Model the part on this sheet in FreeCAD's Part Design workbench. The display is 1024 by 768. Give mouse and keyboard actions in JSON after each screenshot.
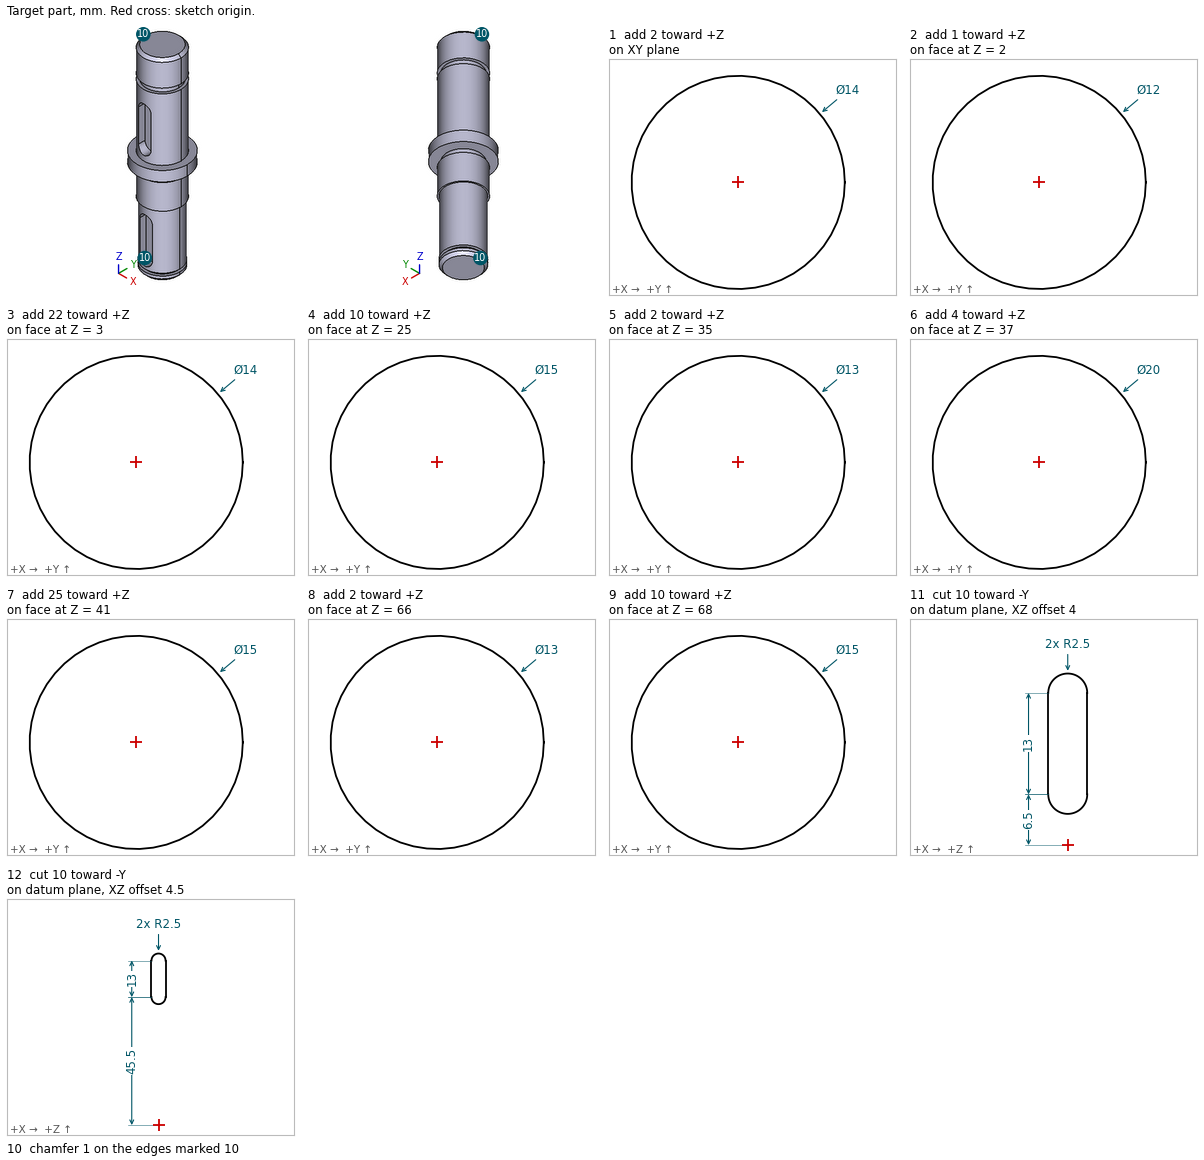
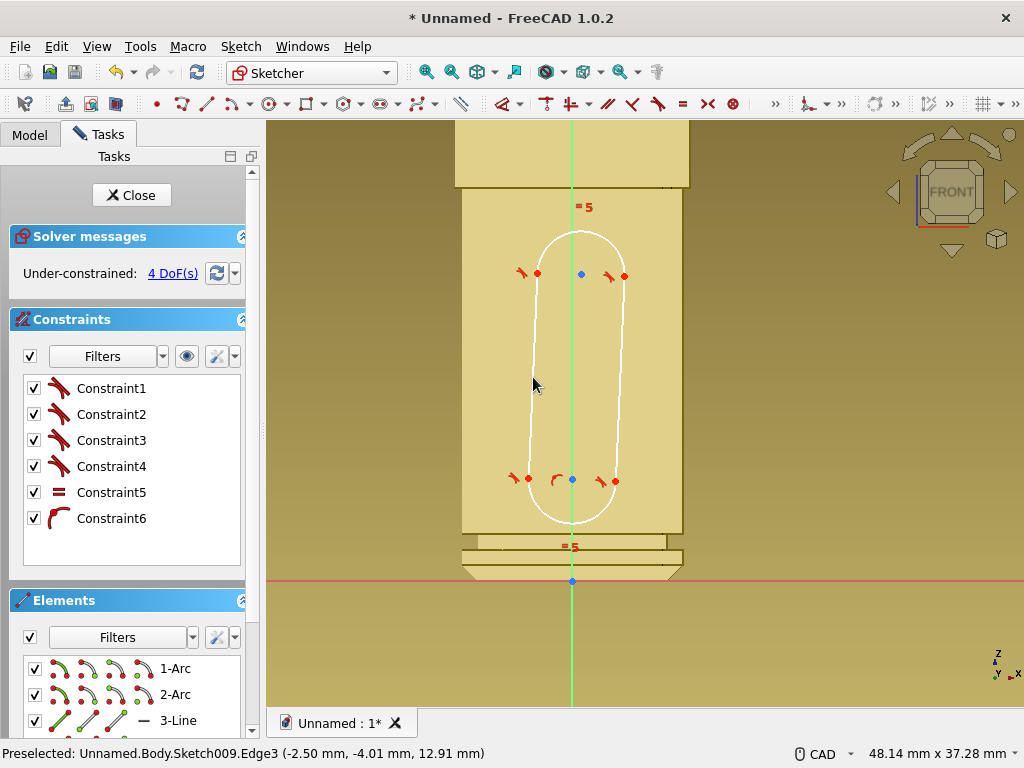
{"action": "left_click", "coordinate": [531, 417]}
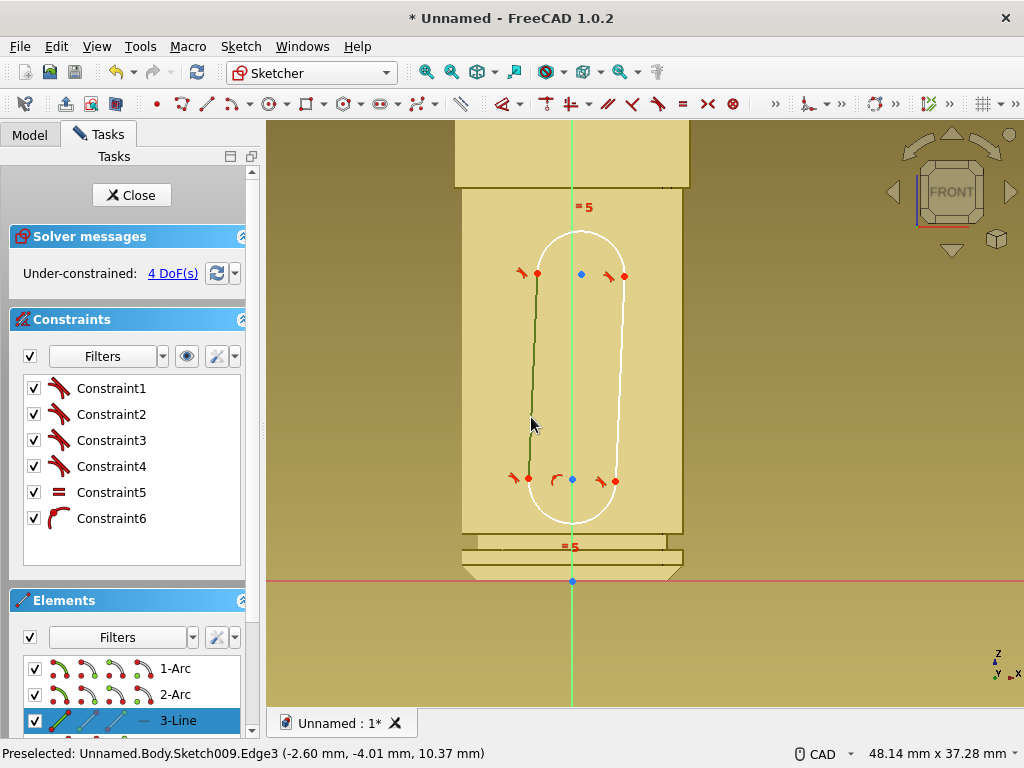
{"action": "left_click", "coordinate": [588, 104]}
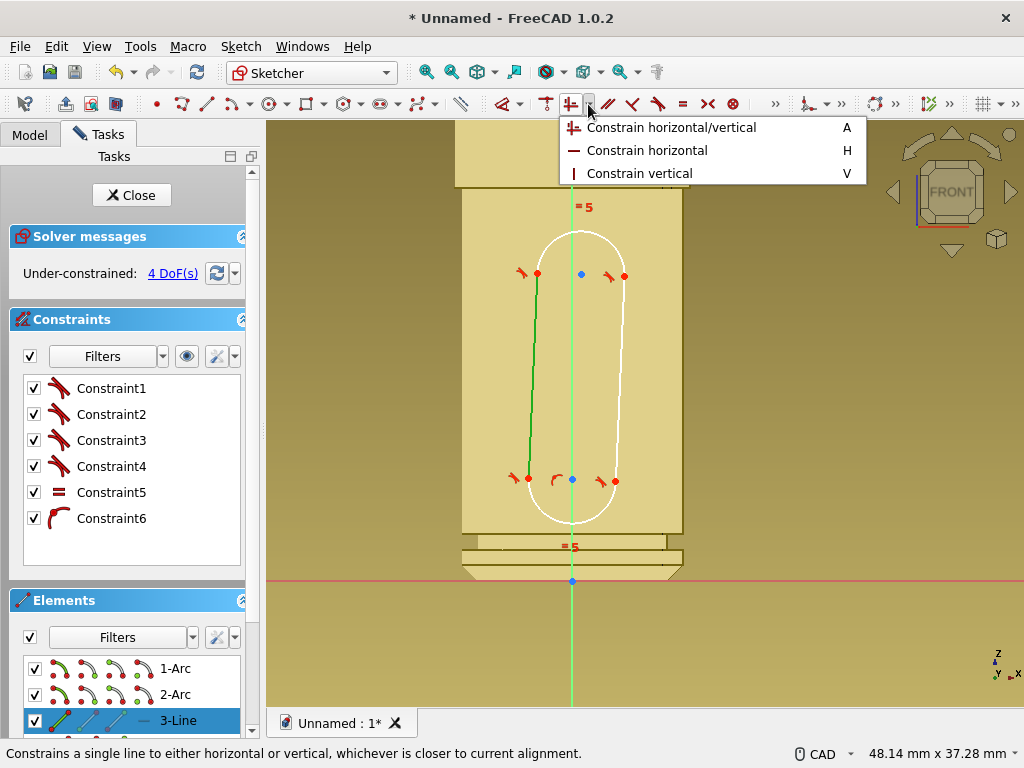
{"action": "left_click", "coordinate": [713, 174]}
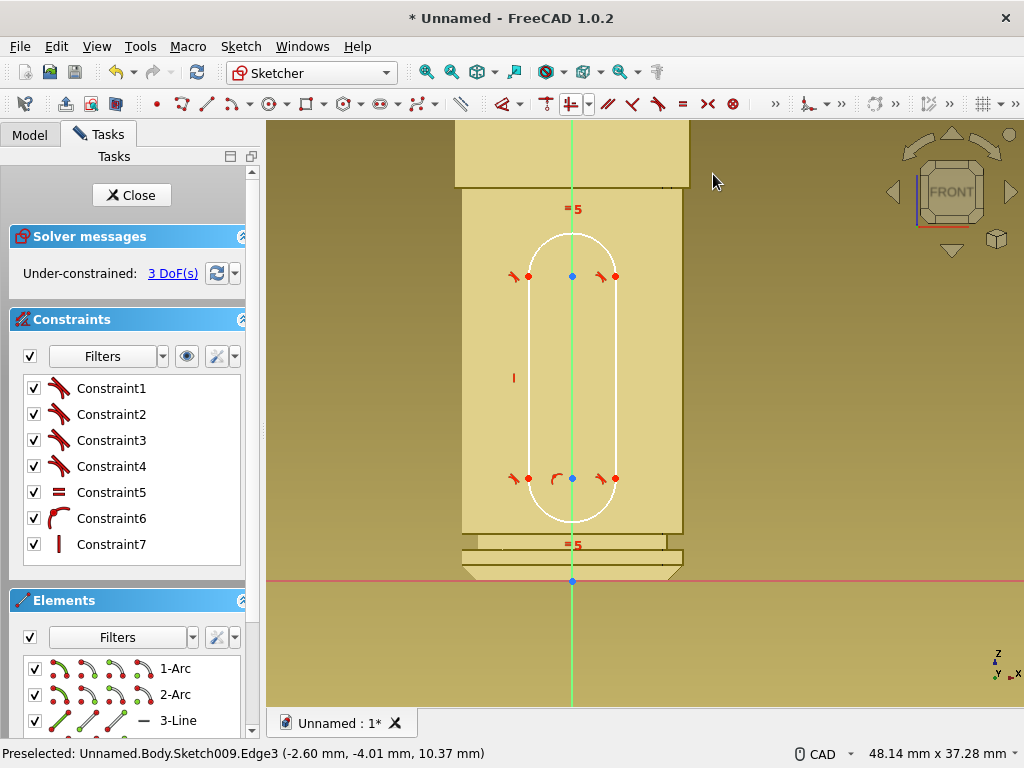
{"action": "left_click", "coordinate": [502, 104]}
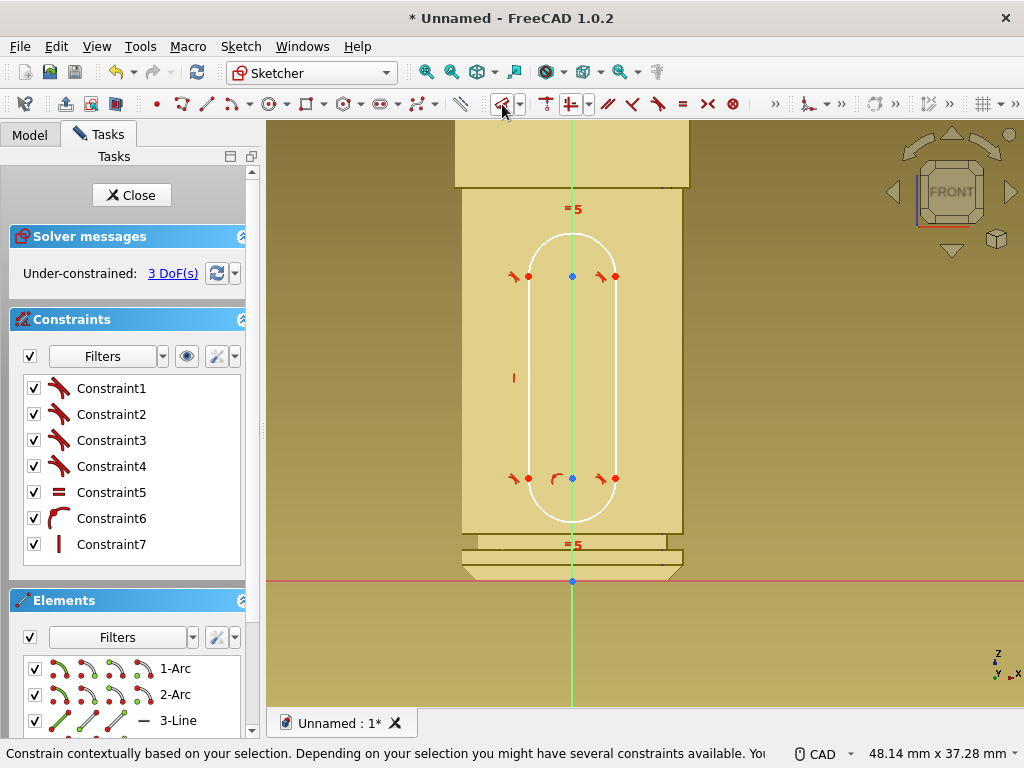
{"action": "left_click", "coordinate": [547, 514]}
{"action": "left_click", "coordinate": [528, 540]}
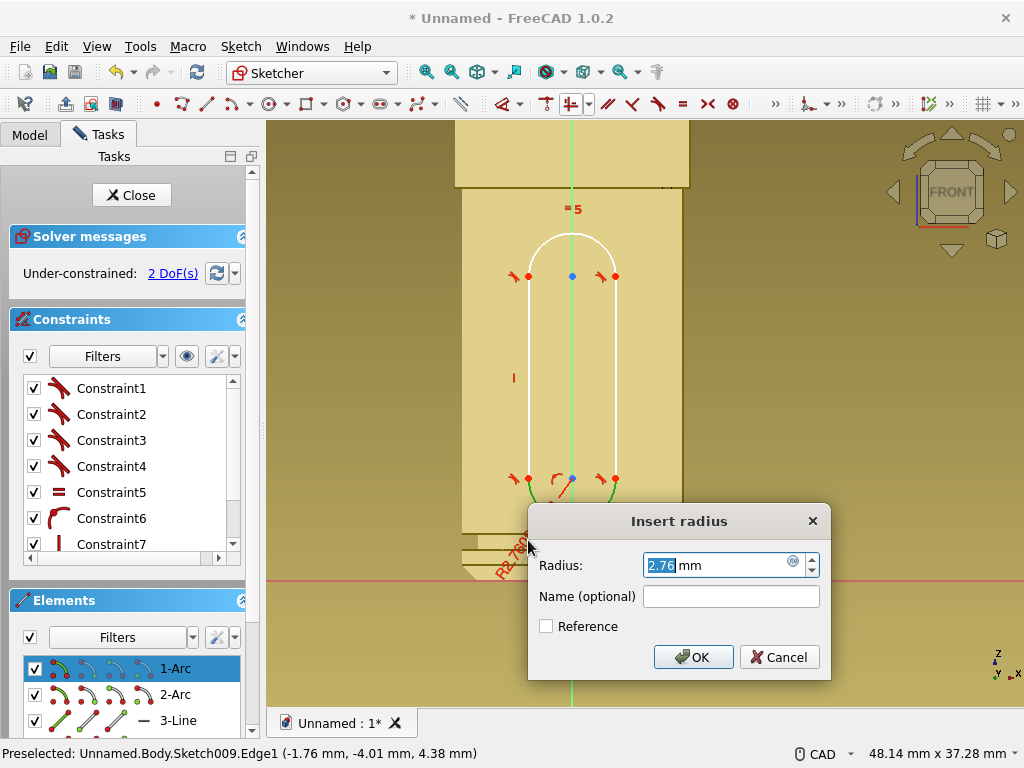
{"action": "type", "text": "2.5"}
{"action": "key", "text": "Return"}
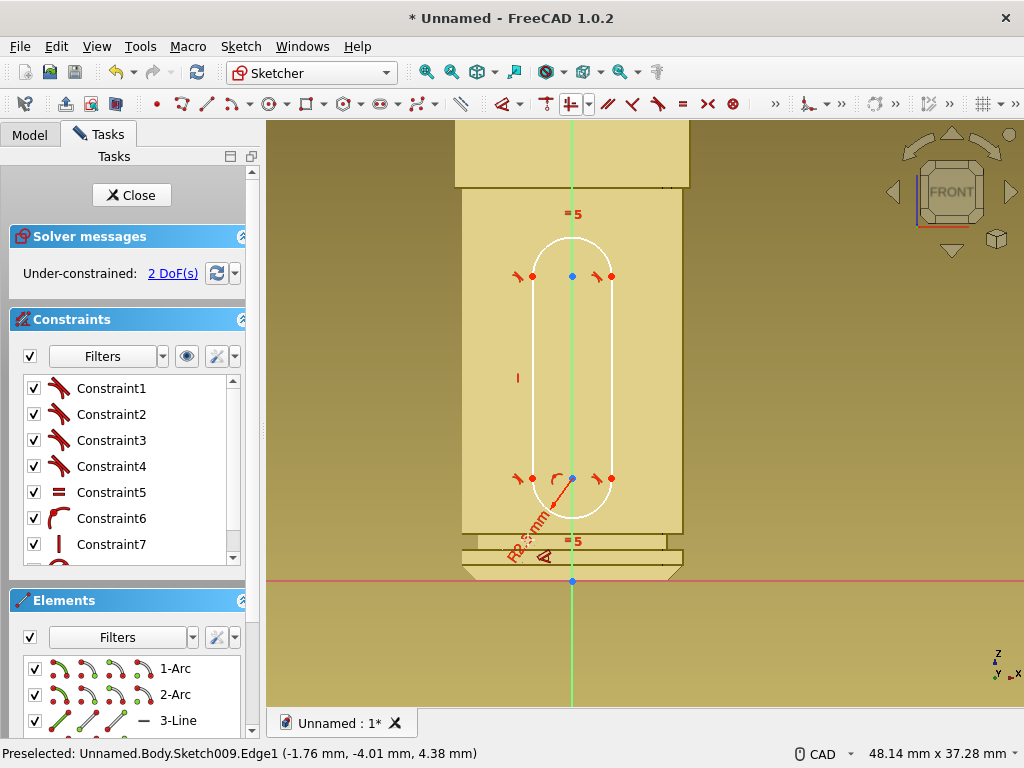
{"action": "left_click", "coordinate": [533, 418]}
{"action": "left_click", "coordinate": [499, 378]}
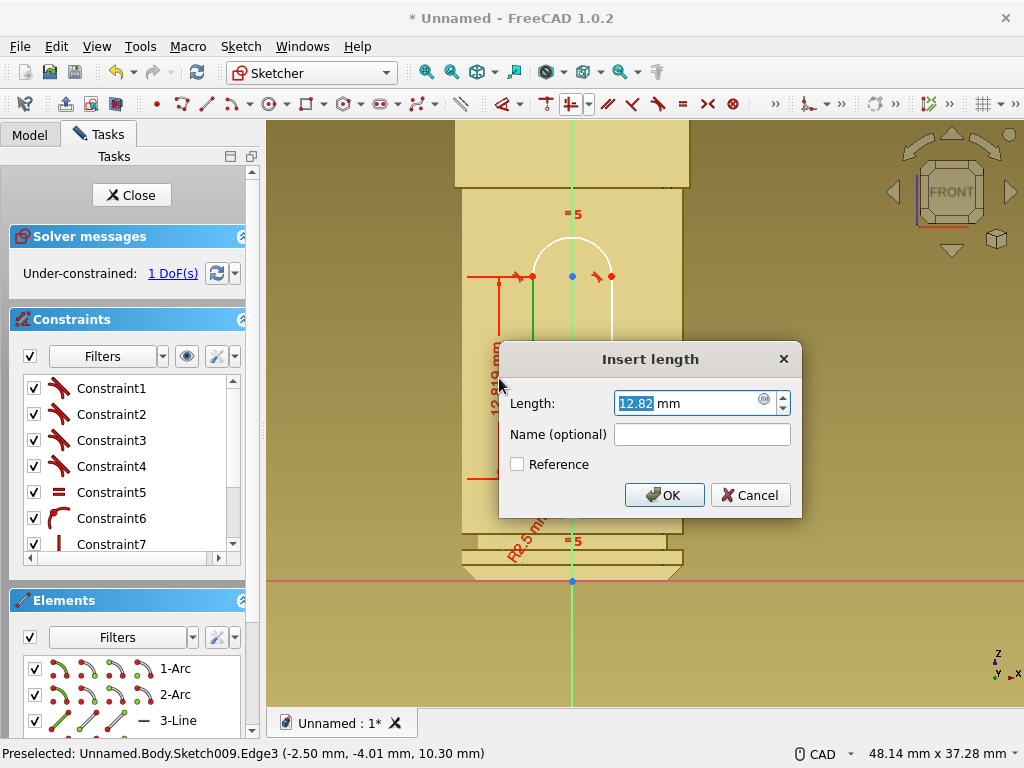
{"action": "type", "text": "13"}
{"action": "key", "text": "Return"}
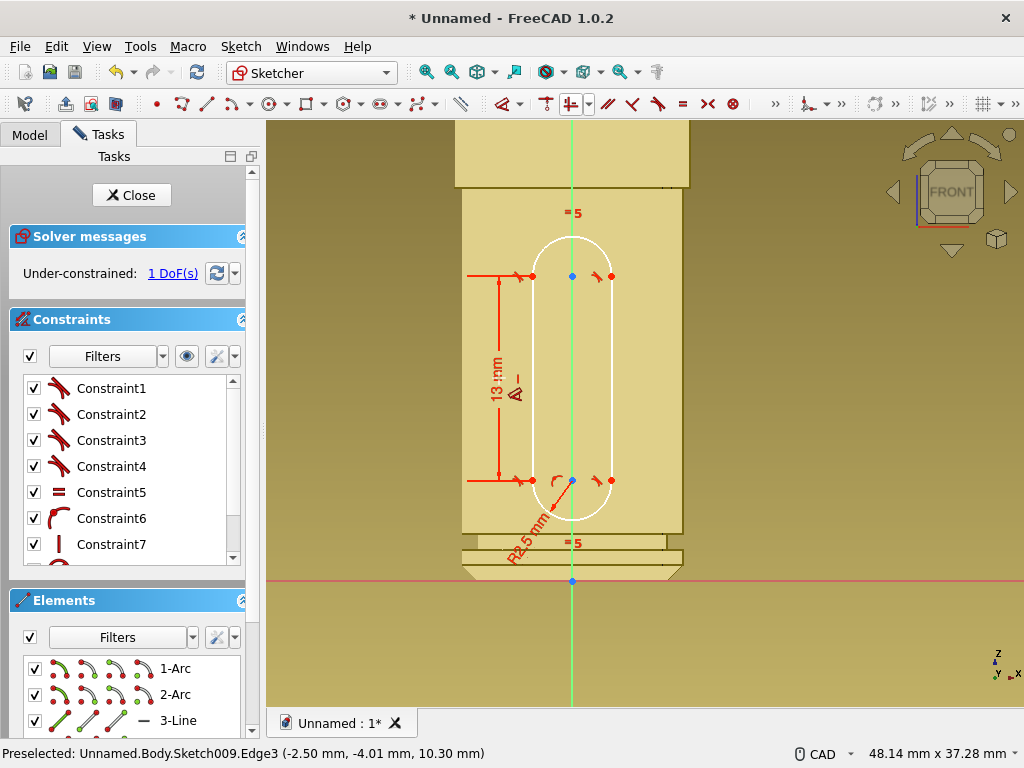
{"action": "left_click", "coordinate": [533, 481]}
{"action": "left_click", "coordinate": [499, 508]}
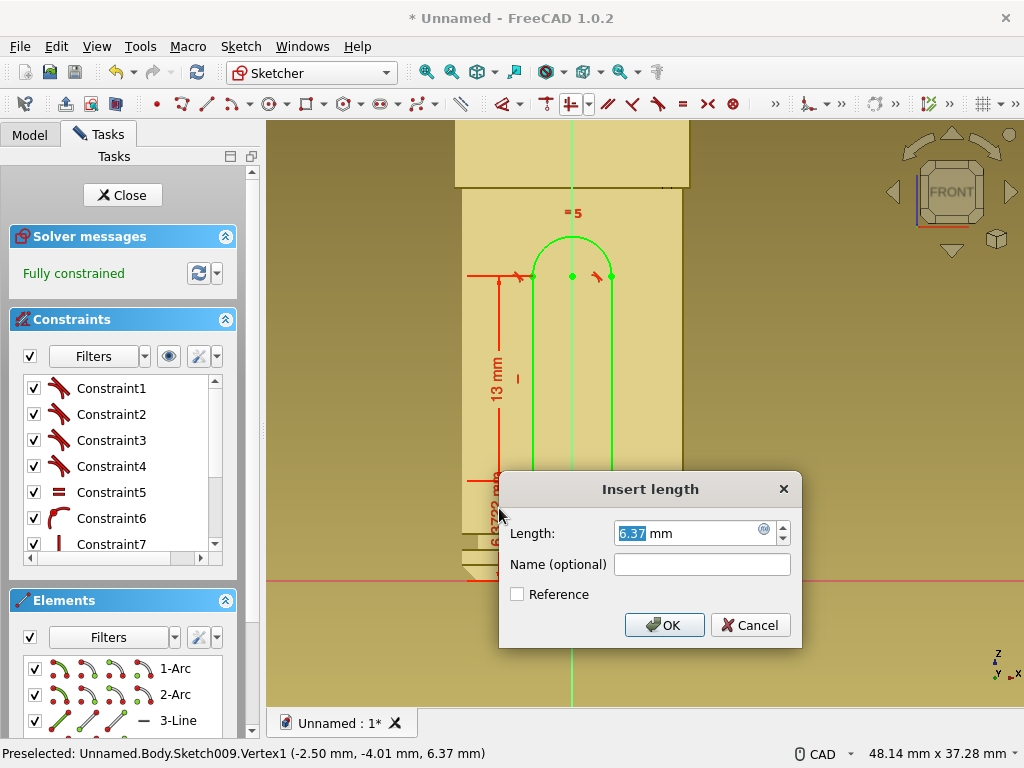
{"action": "type", "text": "6.5"}
{"action": "key", "text": "Return"}
{"action": "key", "text": "Escape"}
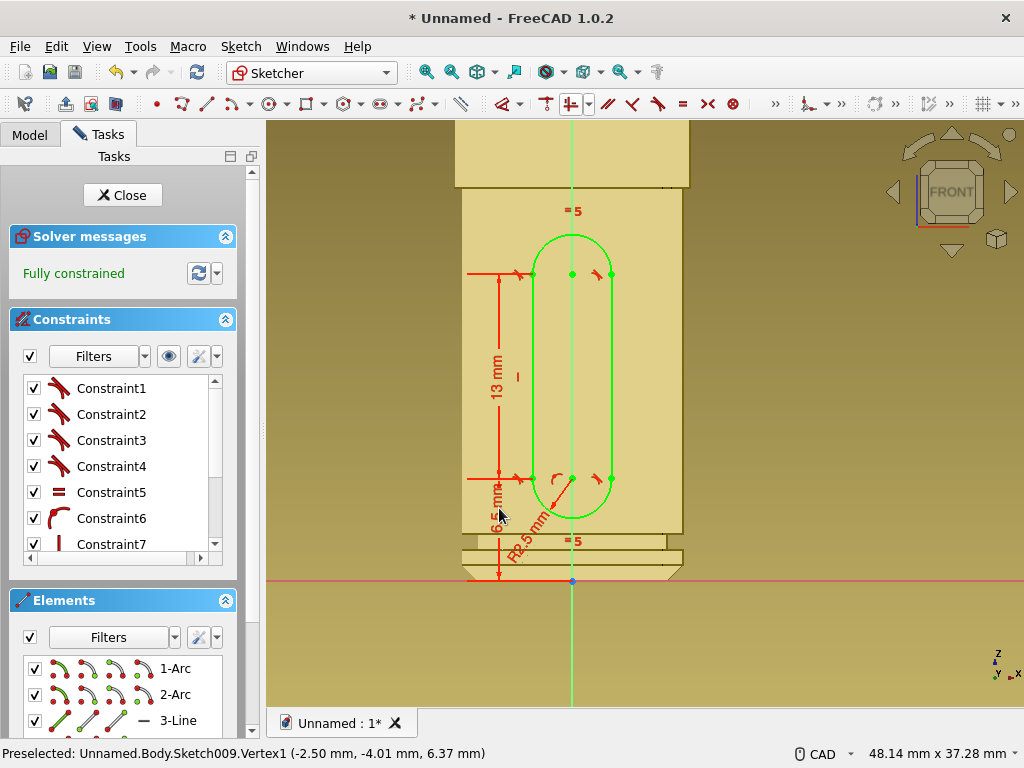
{"action": "left_click", "coordinate": [123, 195]}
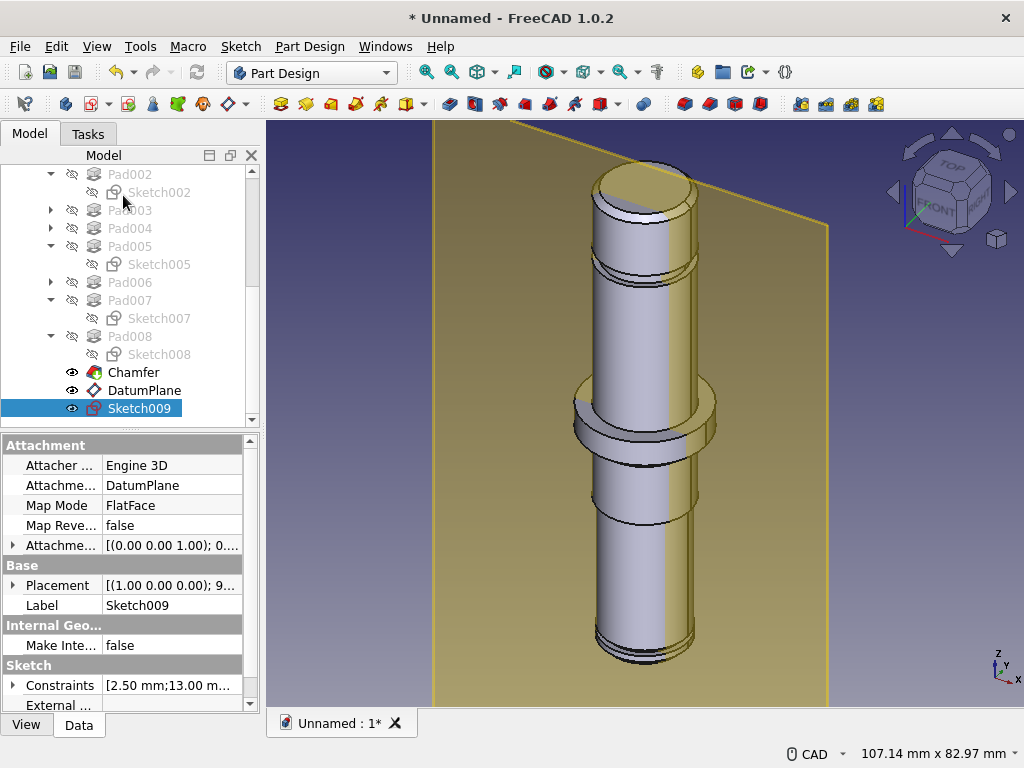
{"action": "left_click", "coordinate": [450, 104]}